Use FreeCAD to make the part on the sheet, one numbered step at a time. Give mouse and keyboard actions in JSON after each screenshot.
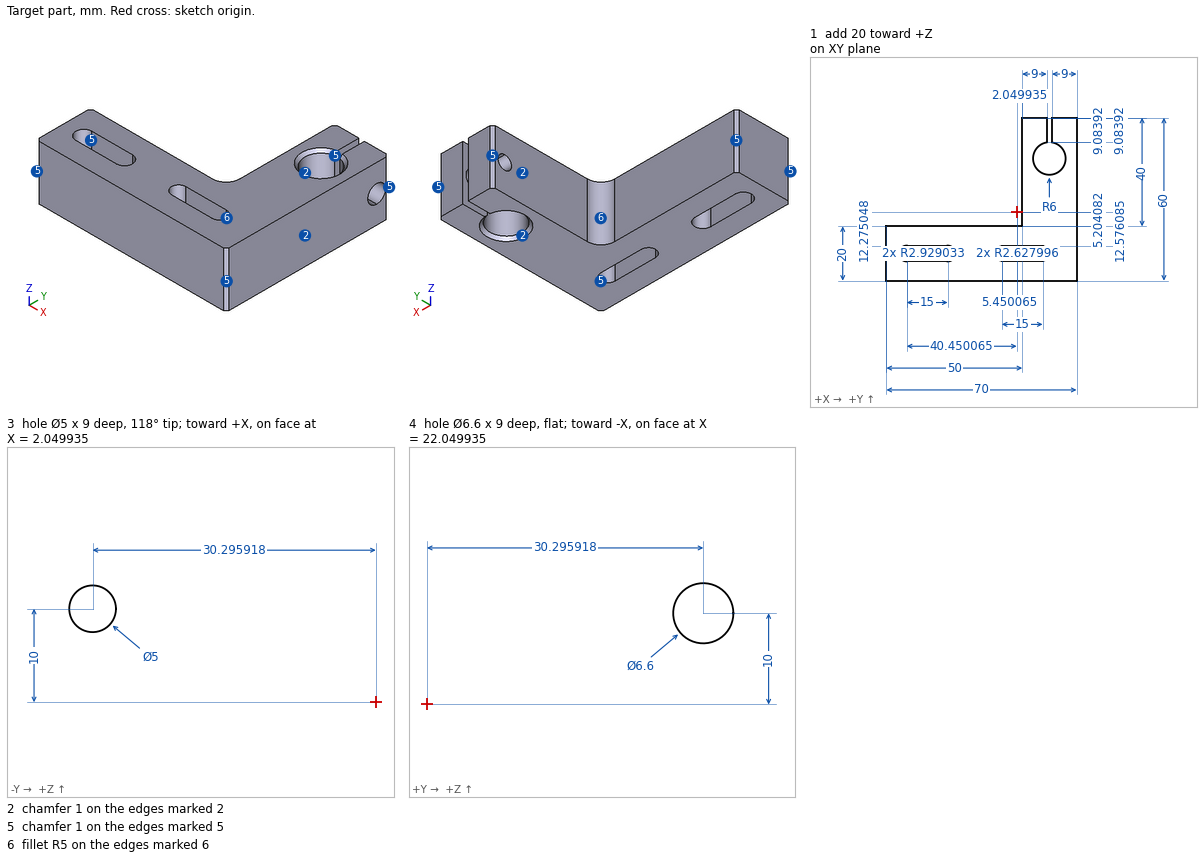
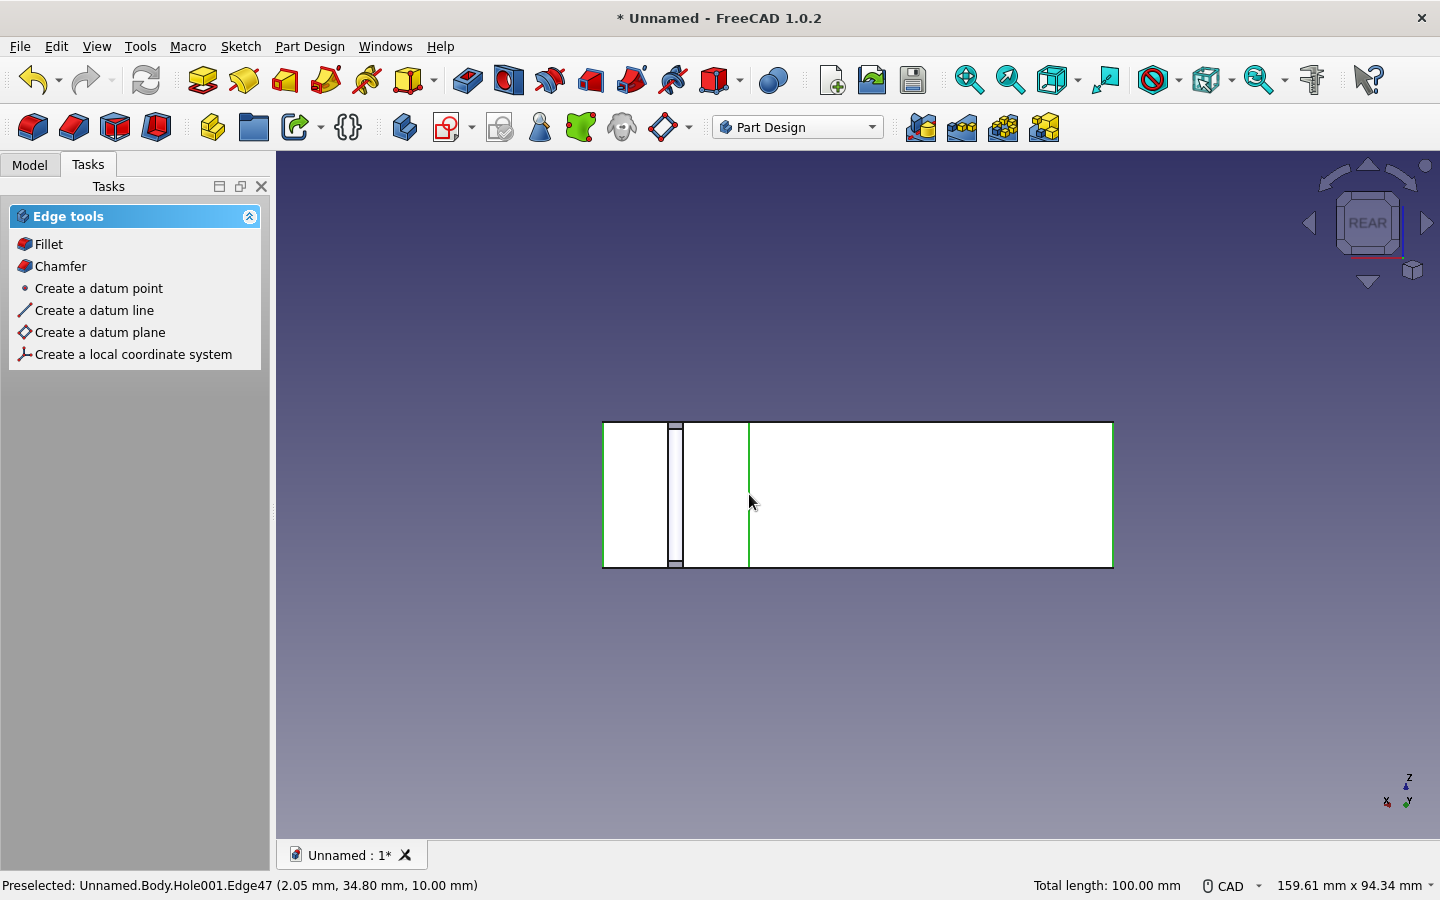
{"action": "left_click", "coordinate": [74, 128]}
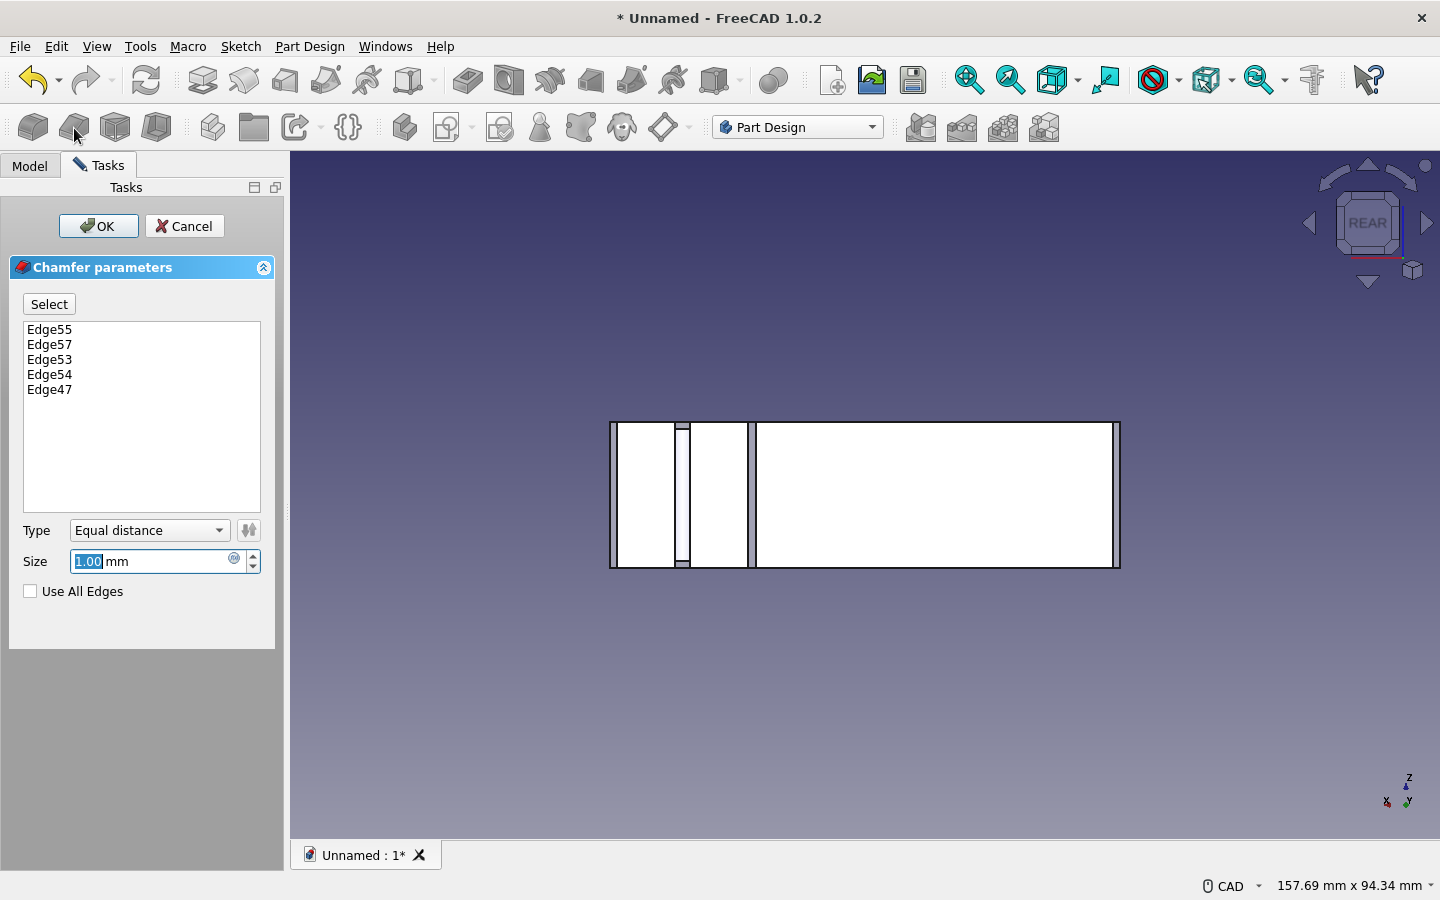
{"action": "type", "text": "1"}
{"action": "key", "text": "Tab"}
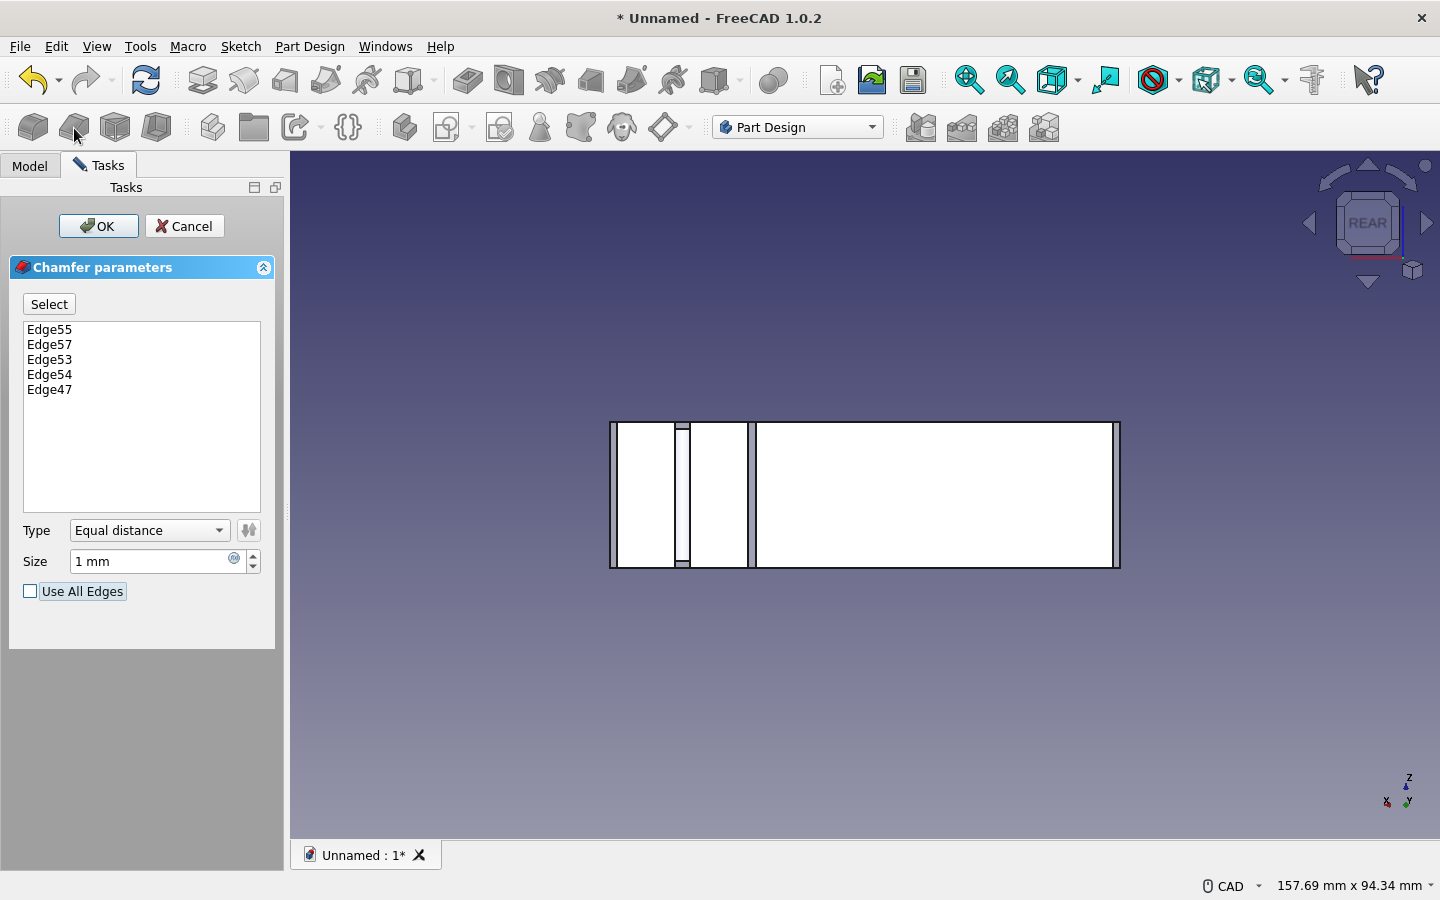
{"action": "left_click", "coordinate": [99, 226]}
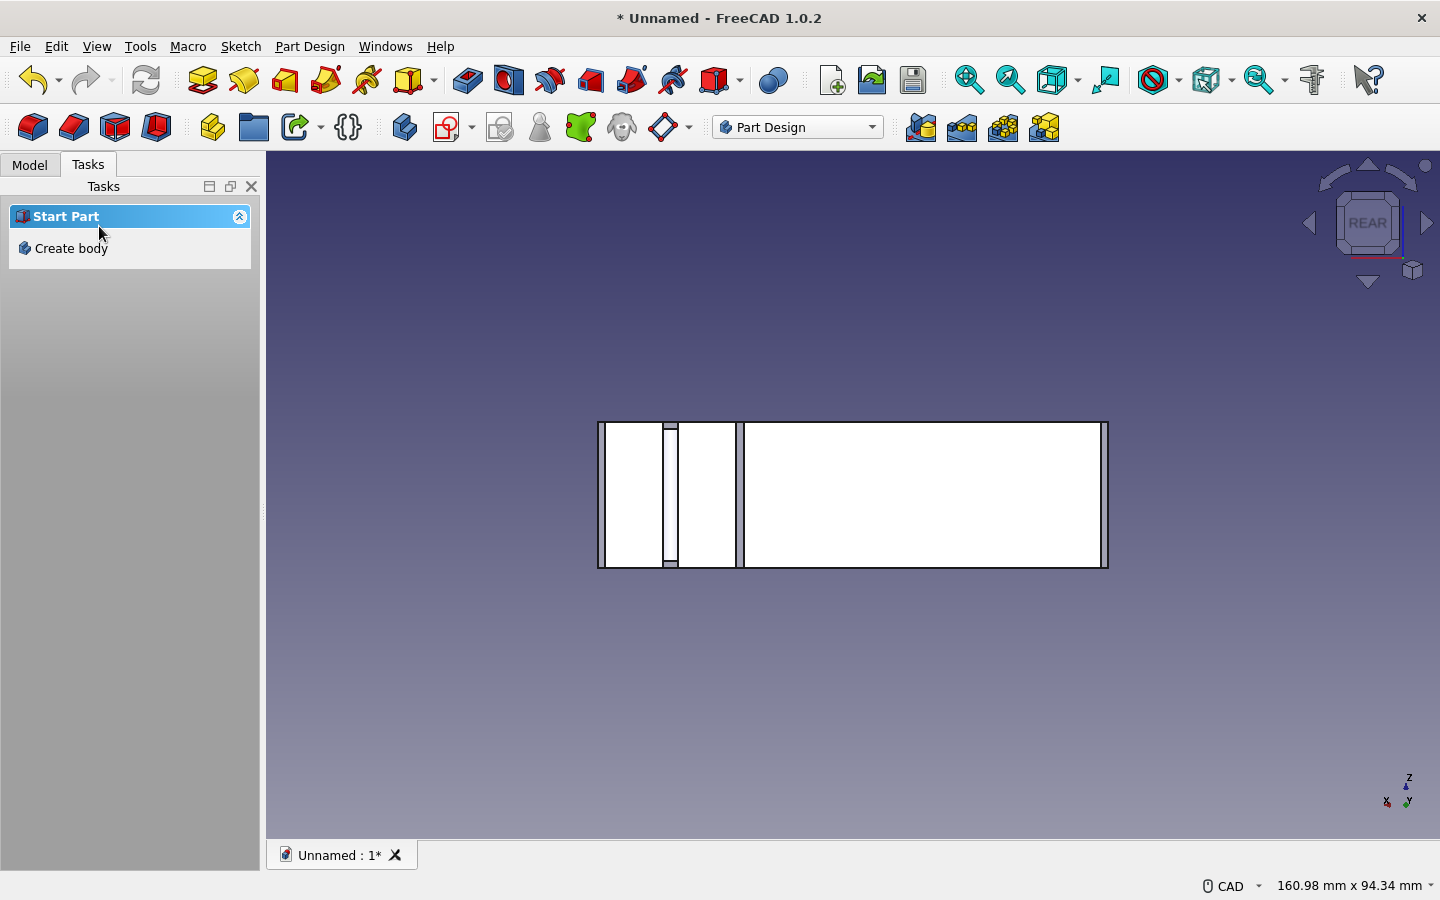
{"action": "left_click", "coordinate": [970, 80]}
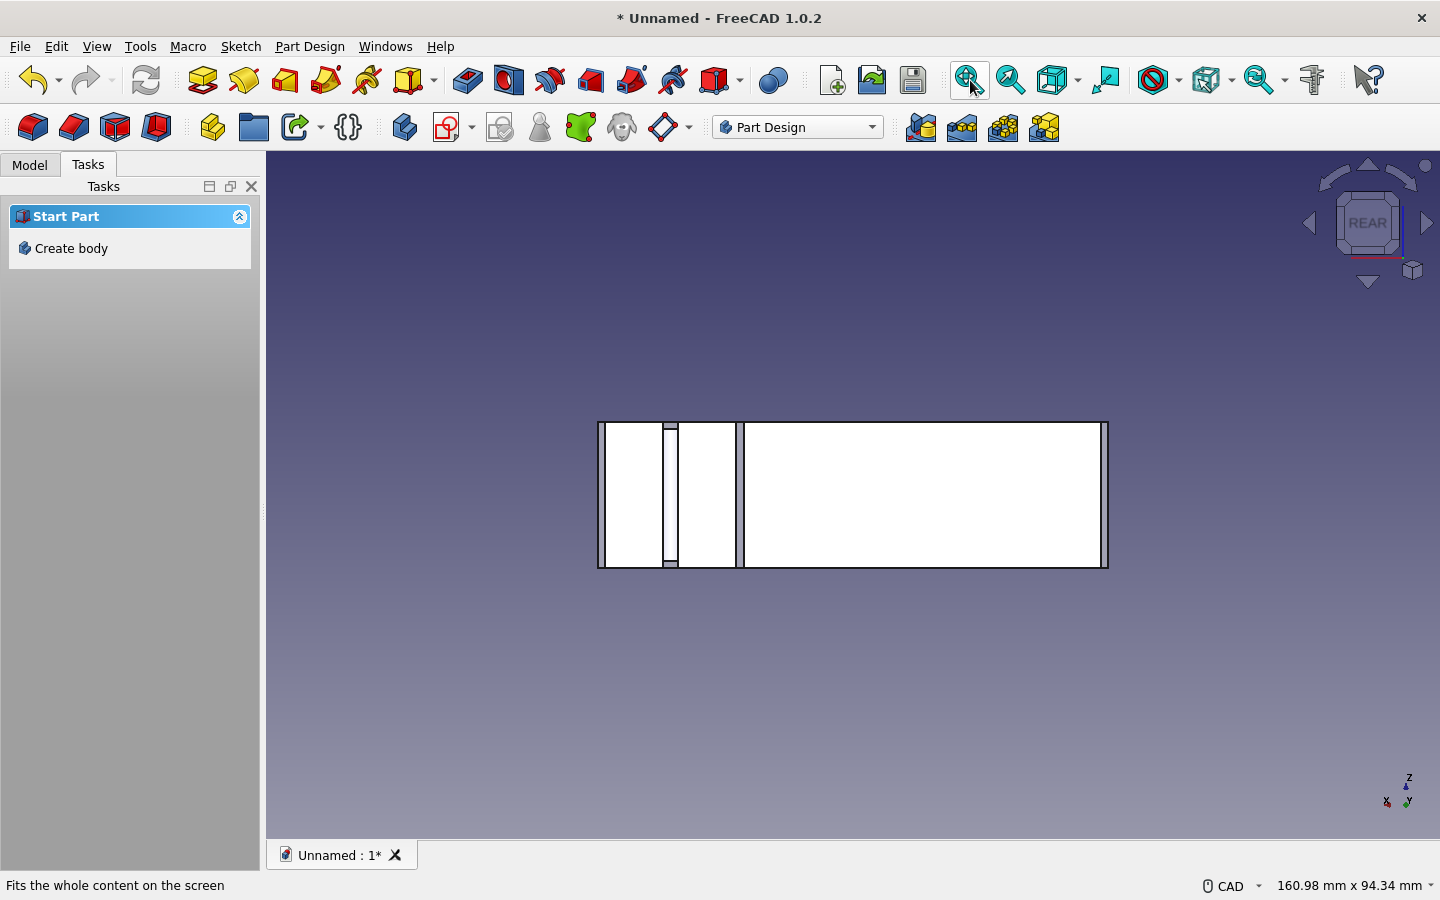
{"action": "key", "text": "0"}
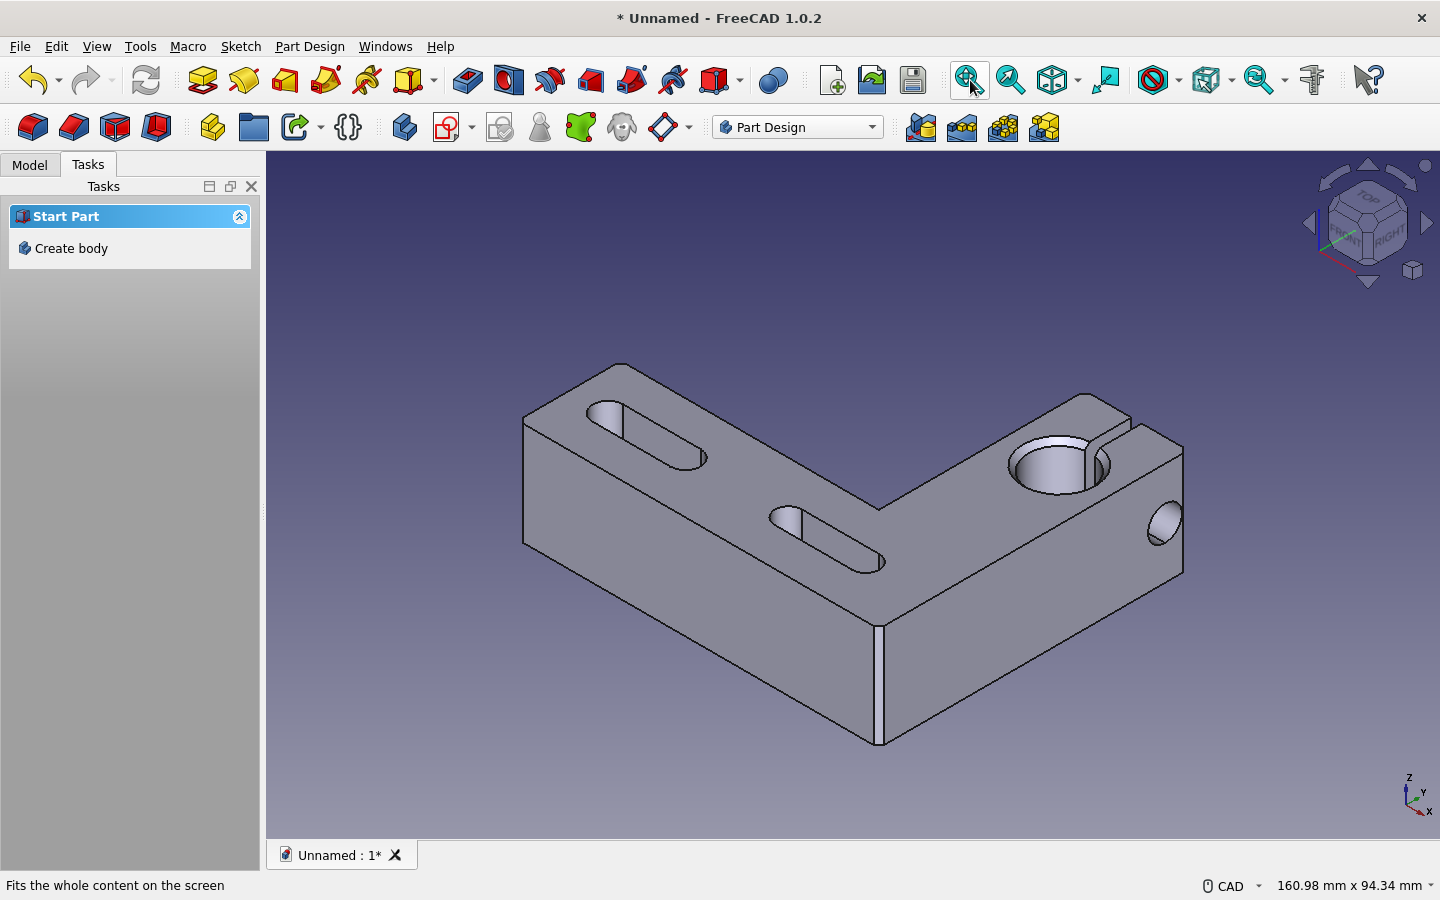
{"action": "key", "text": "2"}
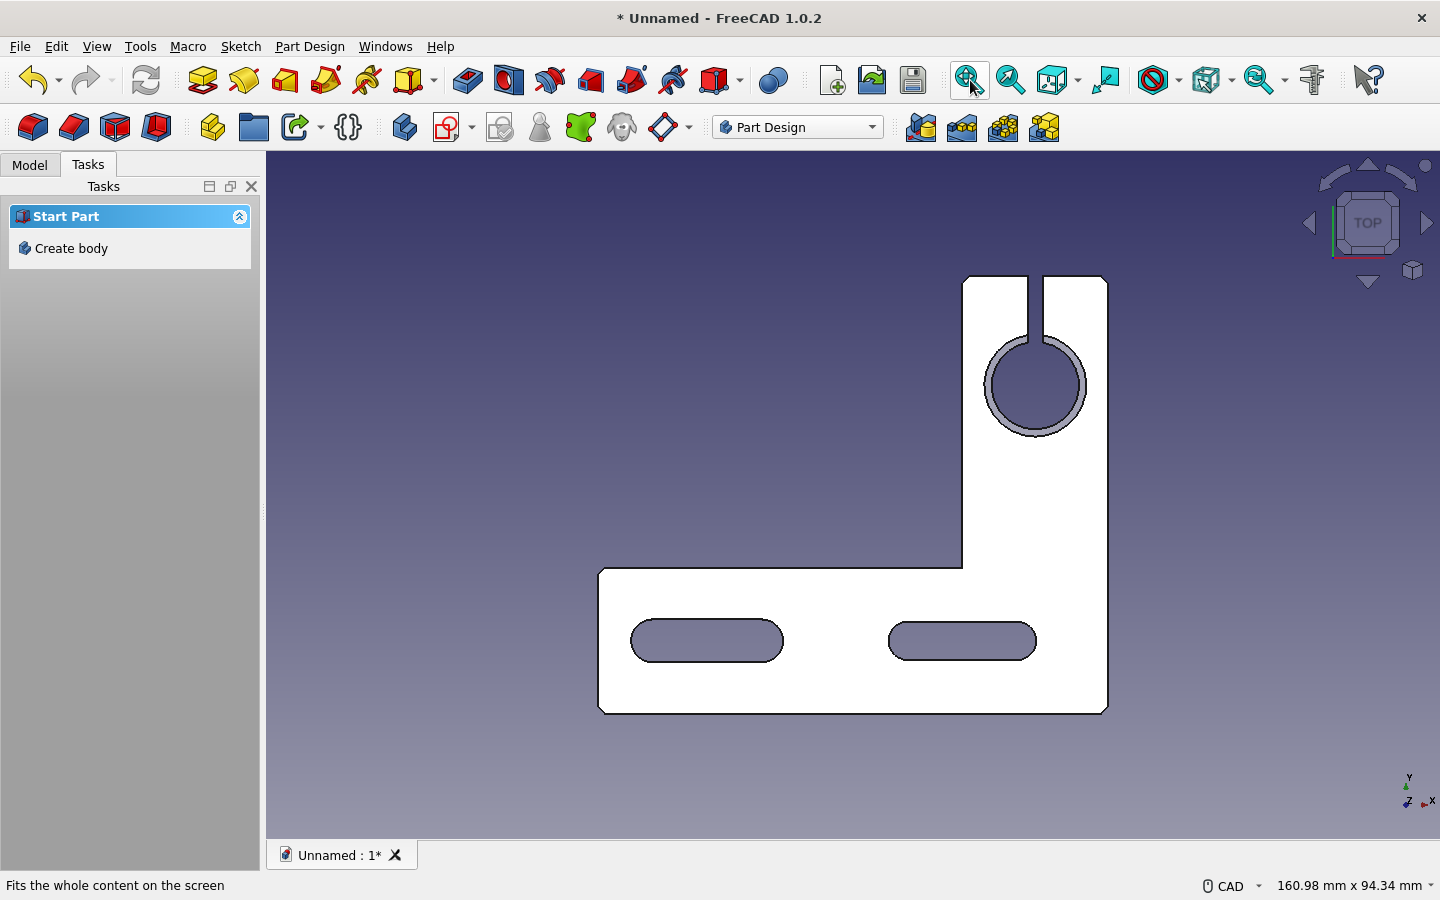
{"action": "key", "text": "1"}